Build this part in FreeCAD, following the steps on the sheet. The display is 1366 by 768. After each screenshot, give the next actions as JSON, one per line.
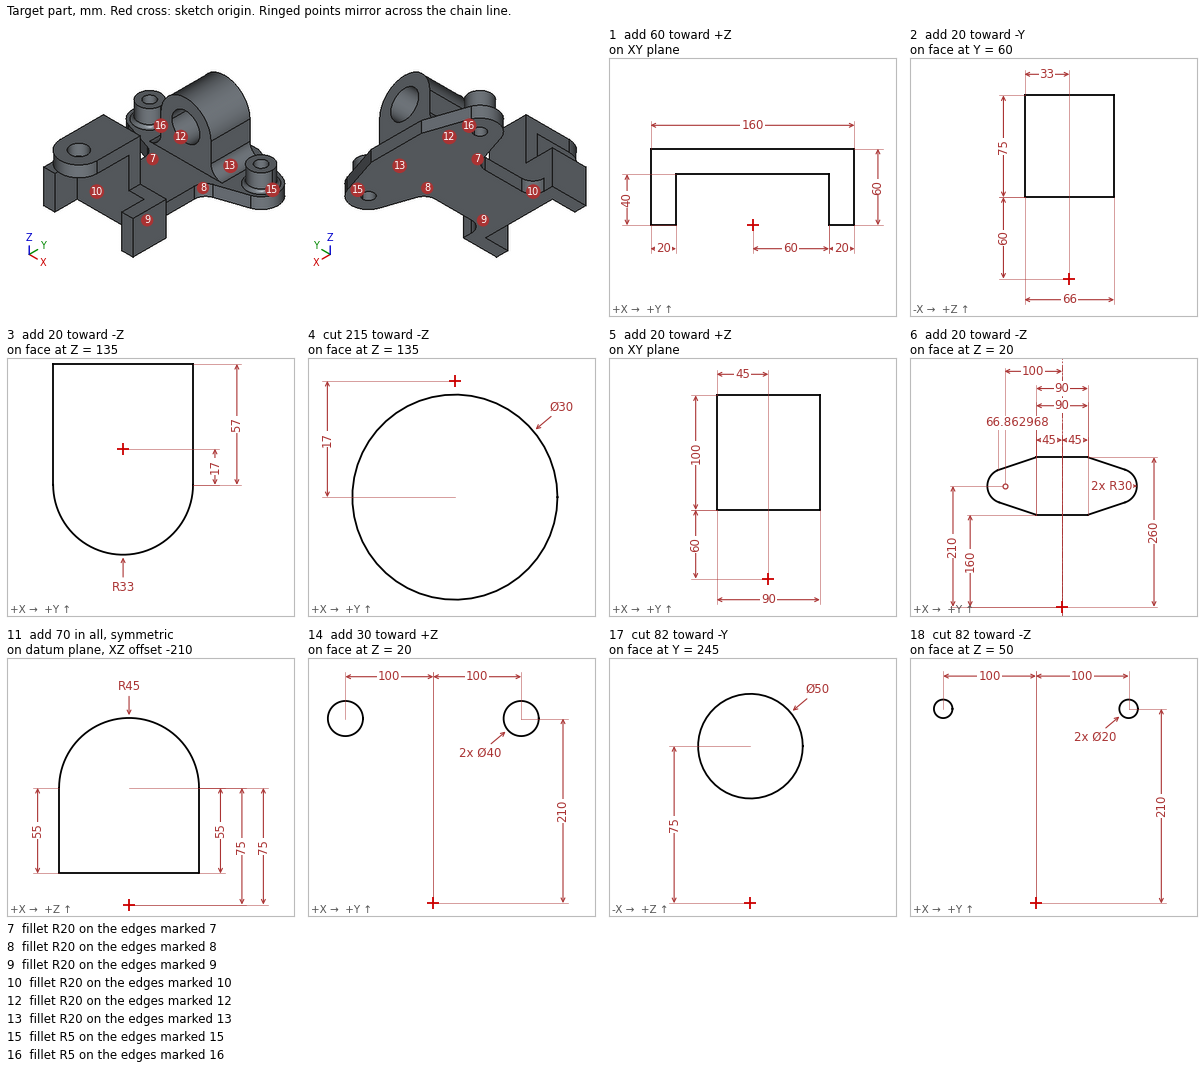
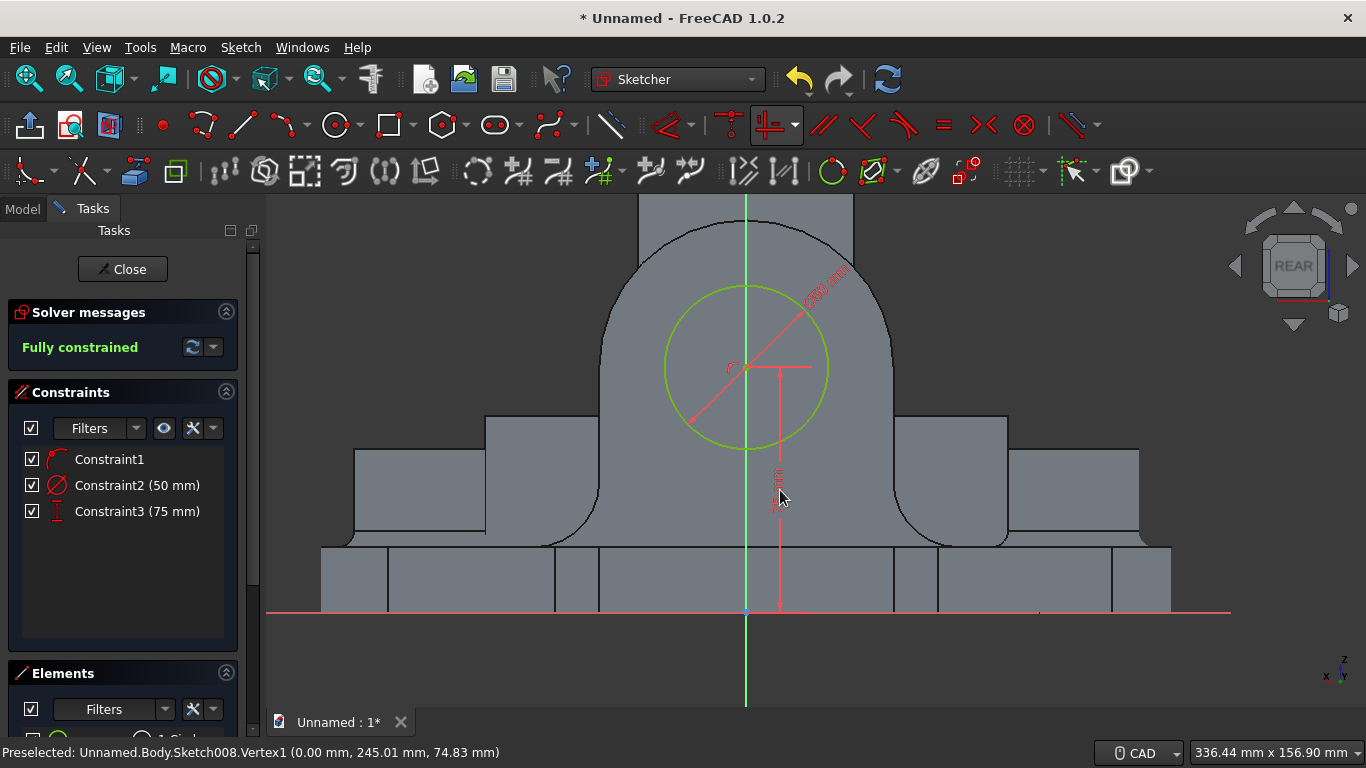
{"action": "left_click", "coordinate": [123, 269]}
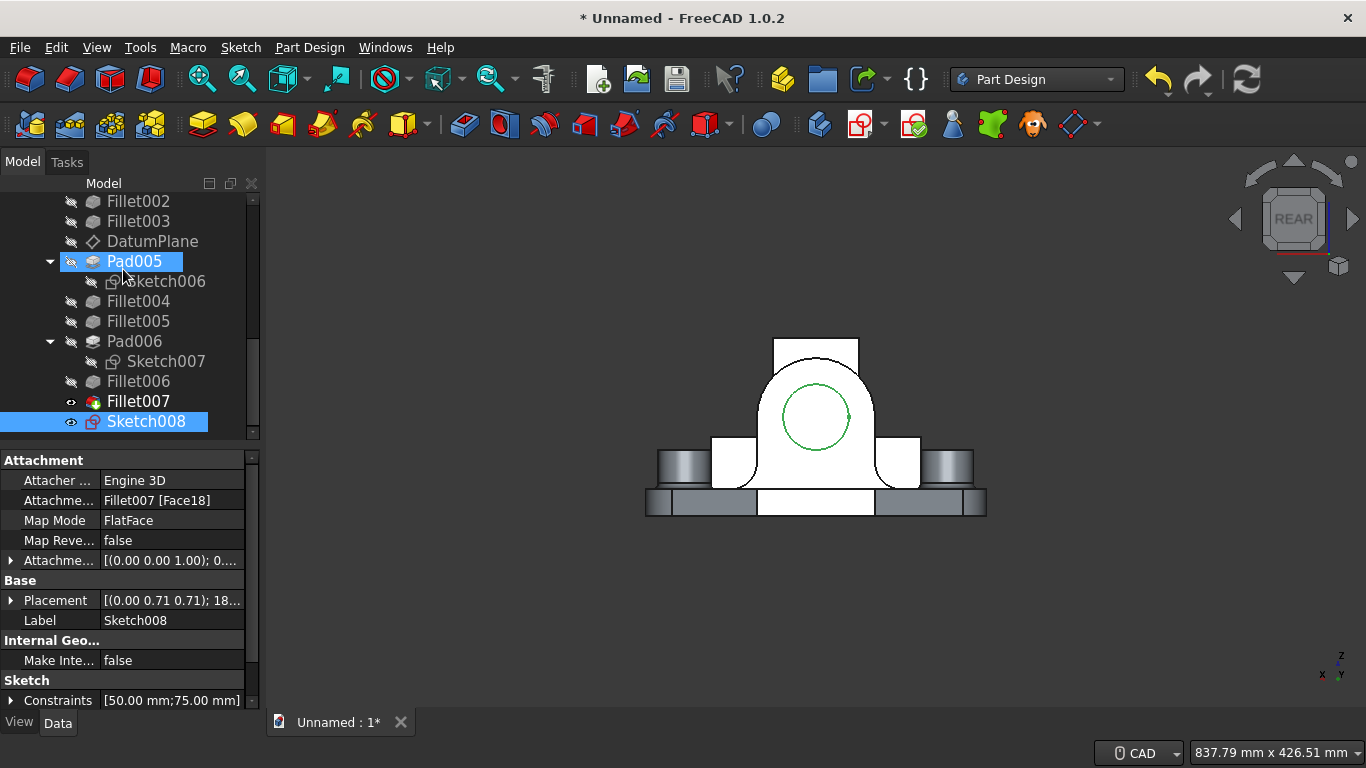
{"action": "left_click", "coordinate": [466, 124]}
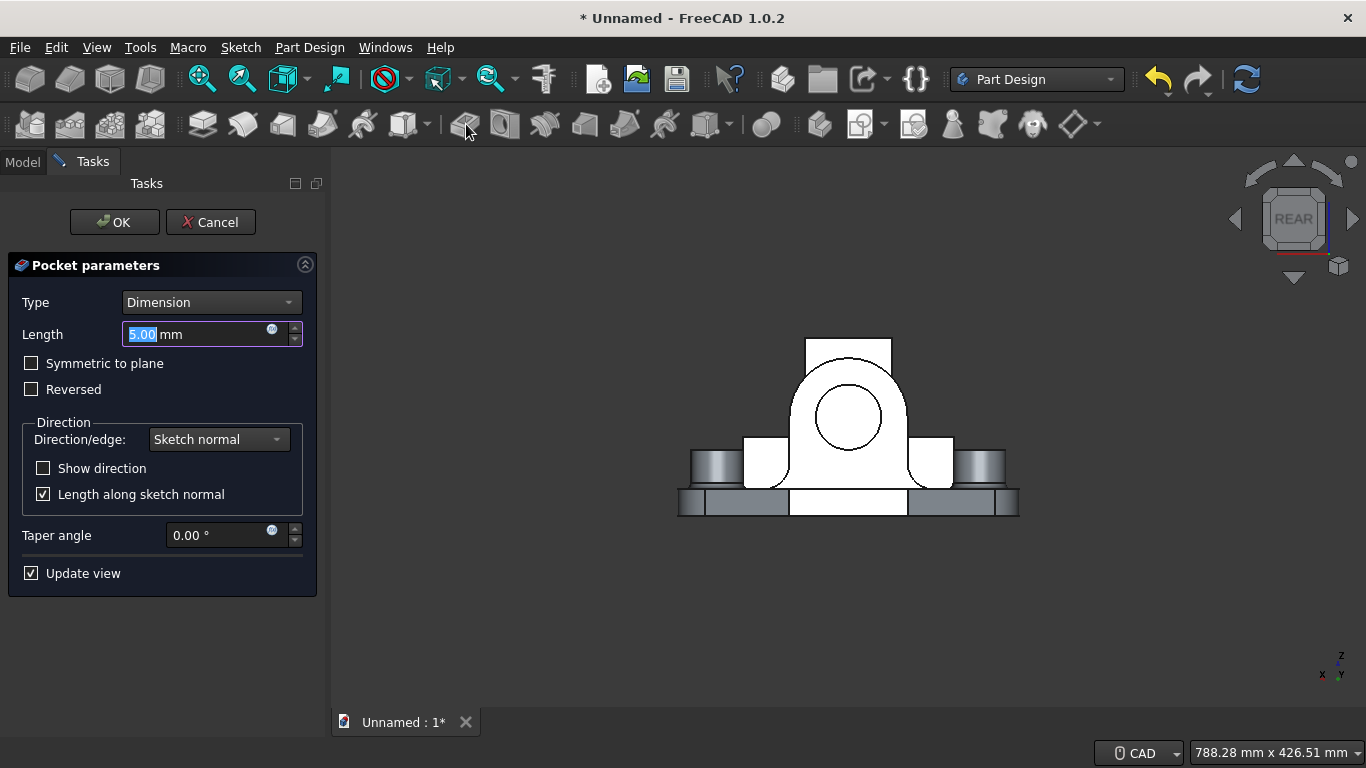
{"action": "type", "text": "82"}
{"action": "key", "text": "Tab"}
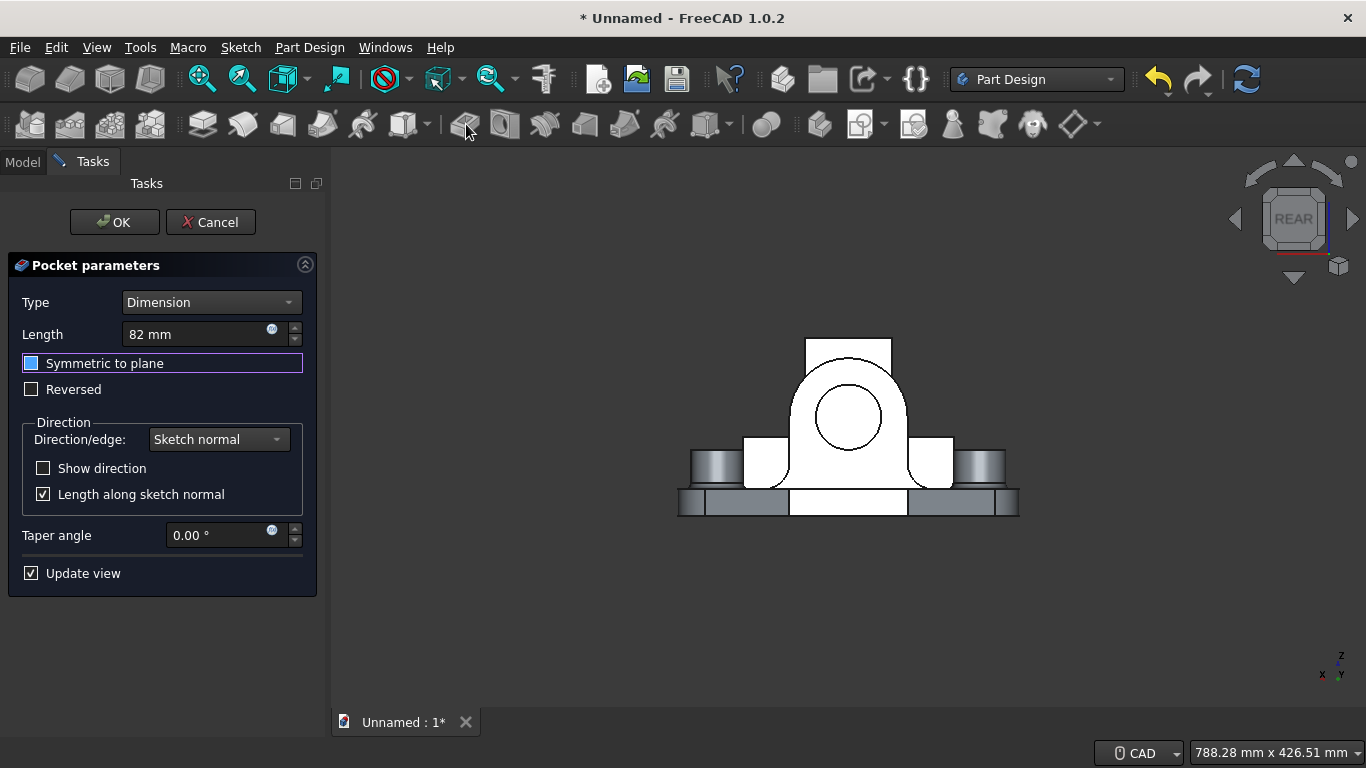
{"action": "left_click", "coordinate": [115, 222]}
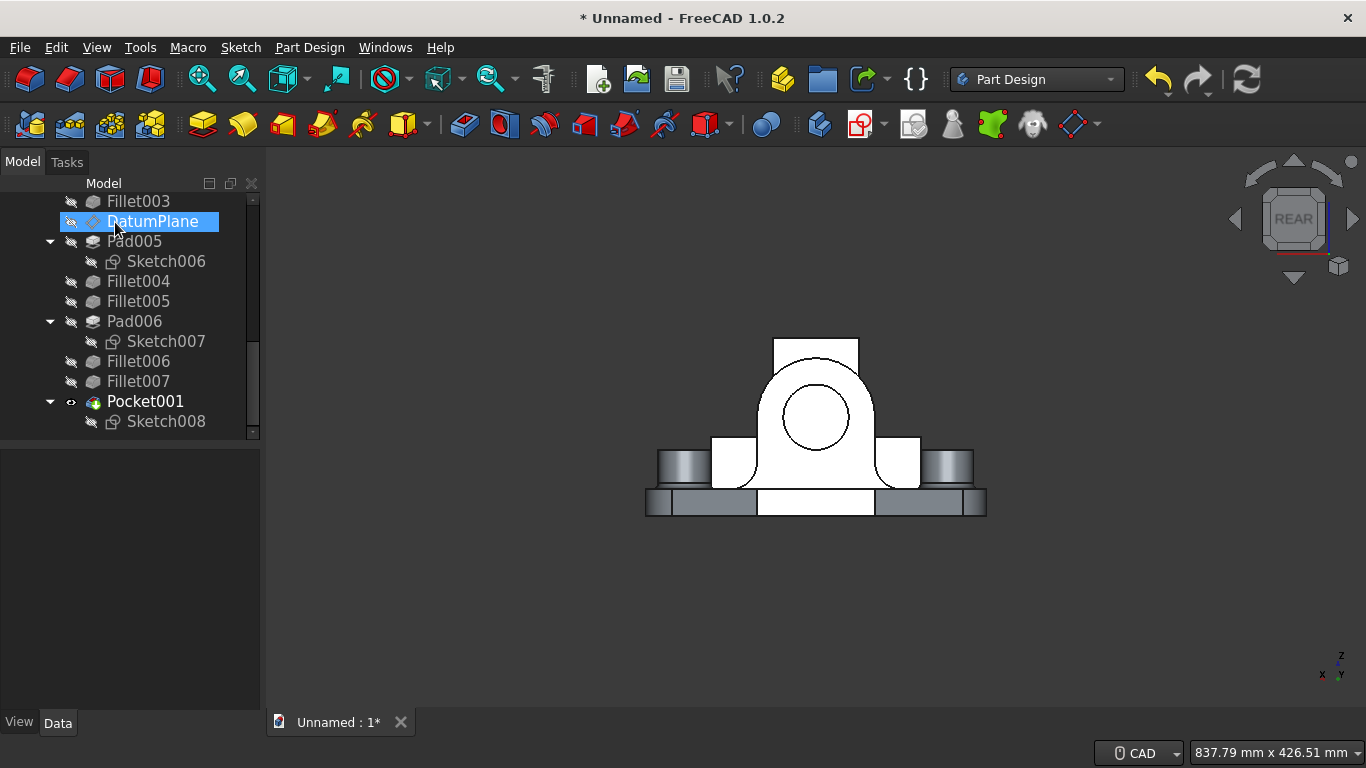
{"action": "key", "text": "v f"}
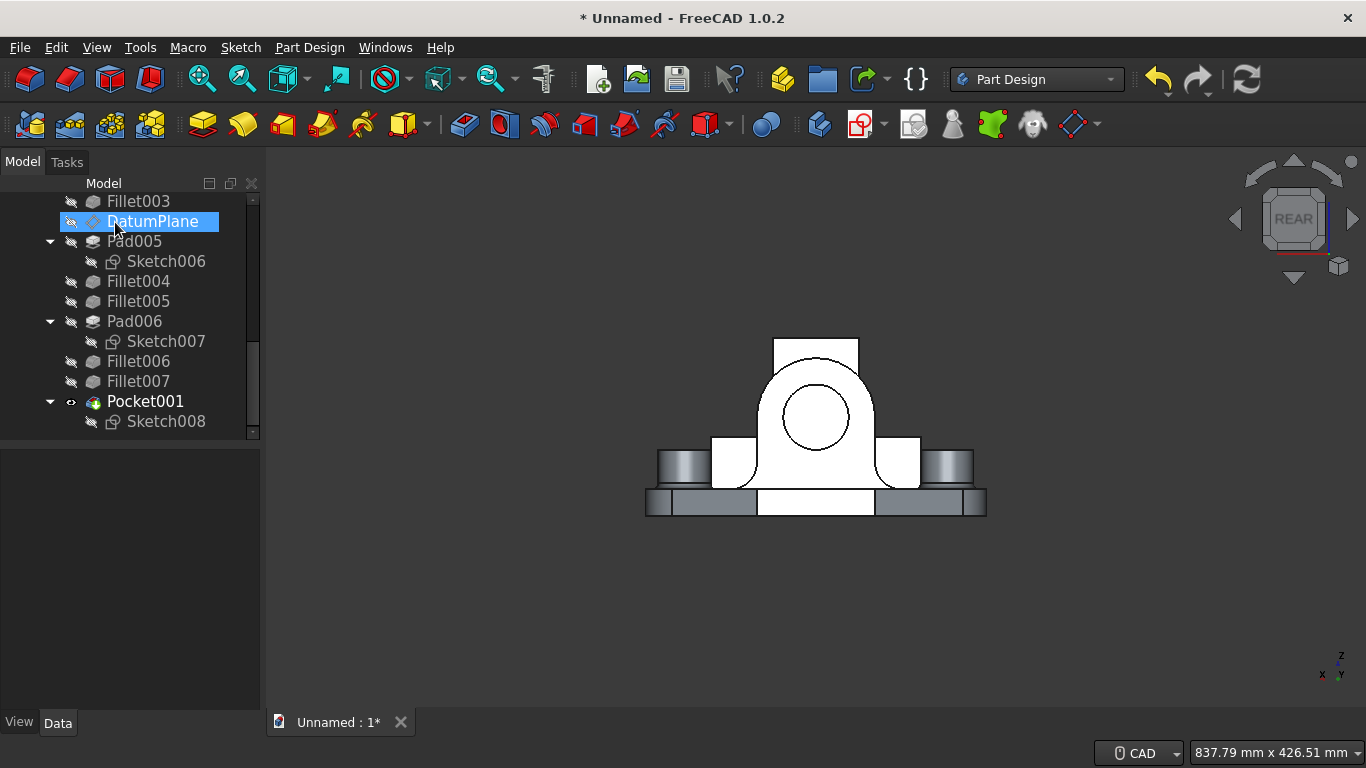
{"action": "key", "text": "0"}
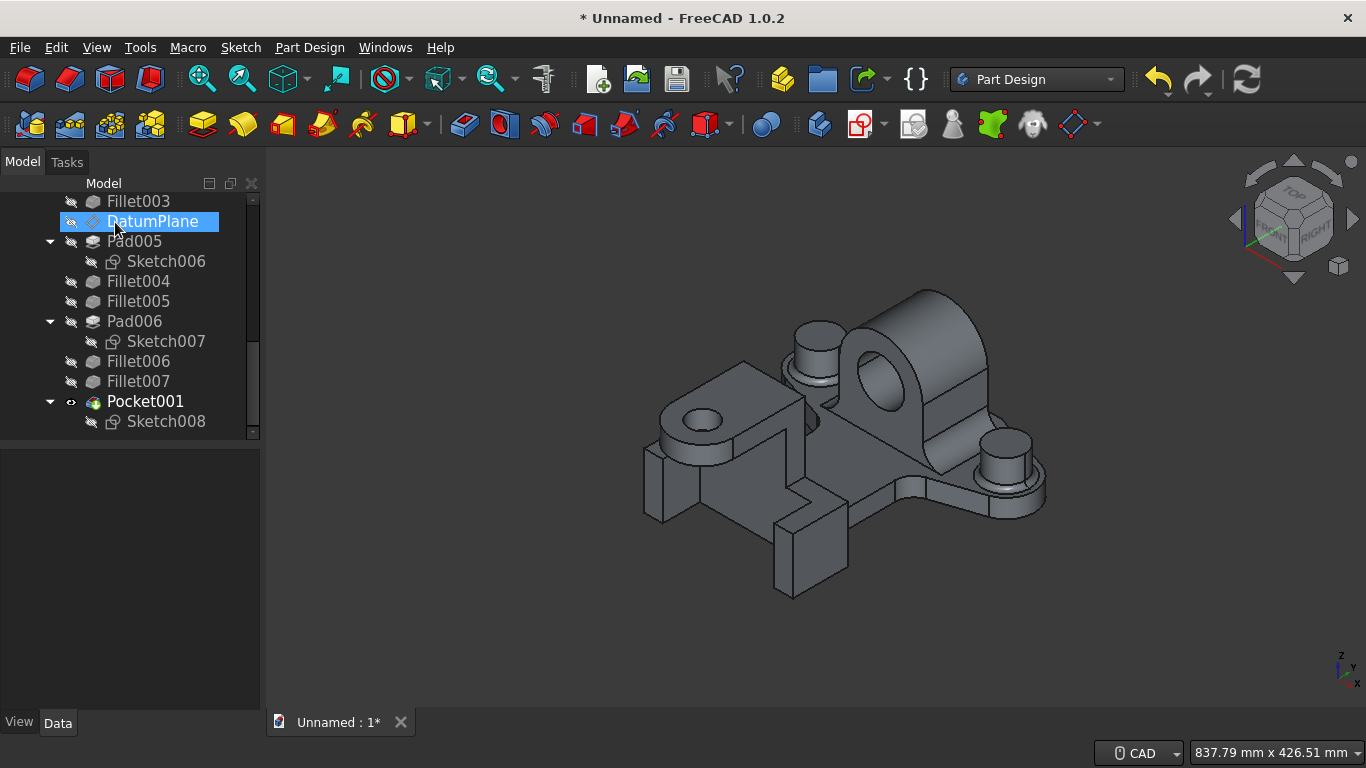
{"action": "left_click", "coordinate": [1006, 442]}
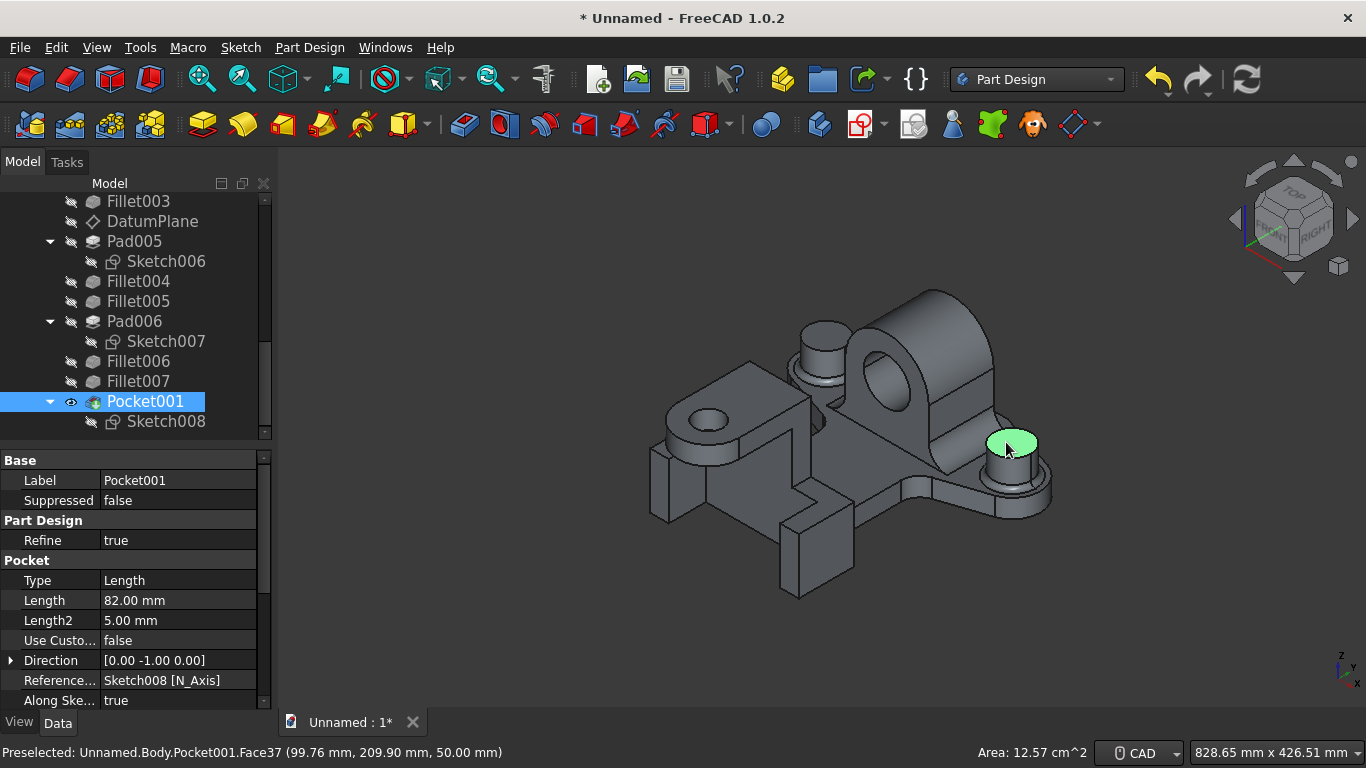
{"action": "left_click", "coordinate": [860, 124]}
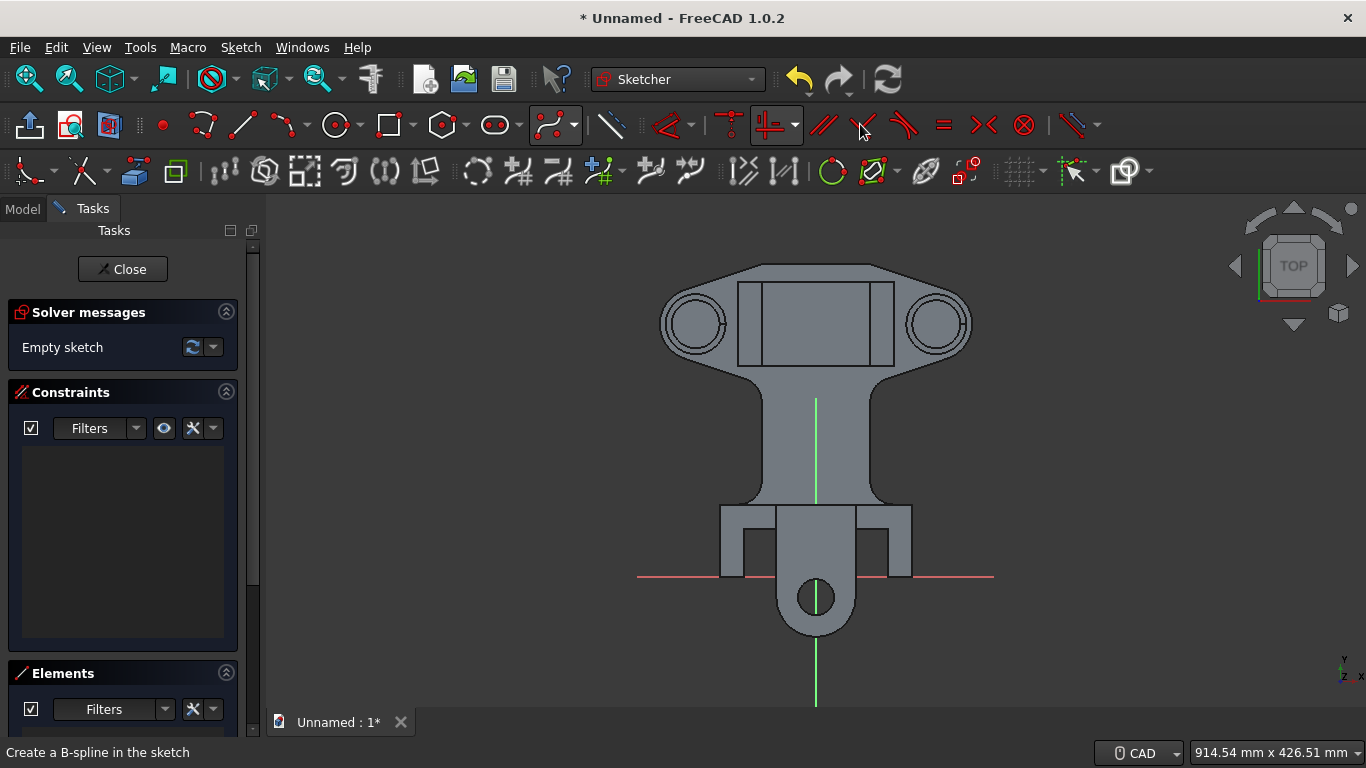
{"action": "left_click", "coordinate": [336, 126]}